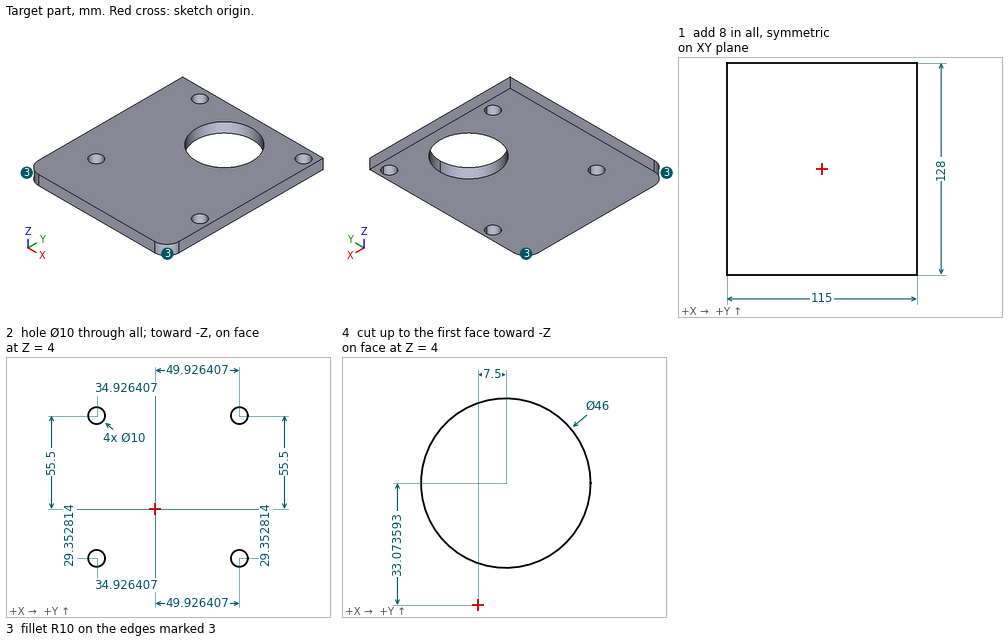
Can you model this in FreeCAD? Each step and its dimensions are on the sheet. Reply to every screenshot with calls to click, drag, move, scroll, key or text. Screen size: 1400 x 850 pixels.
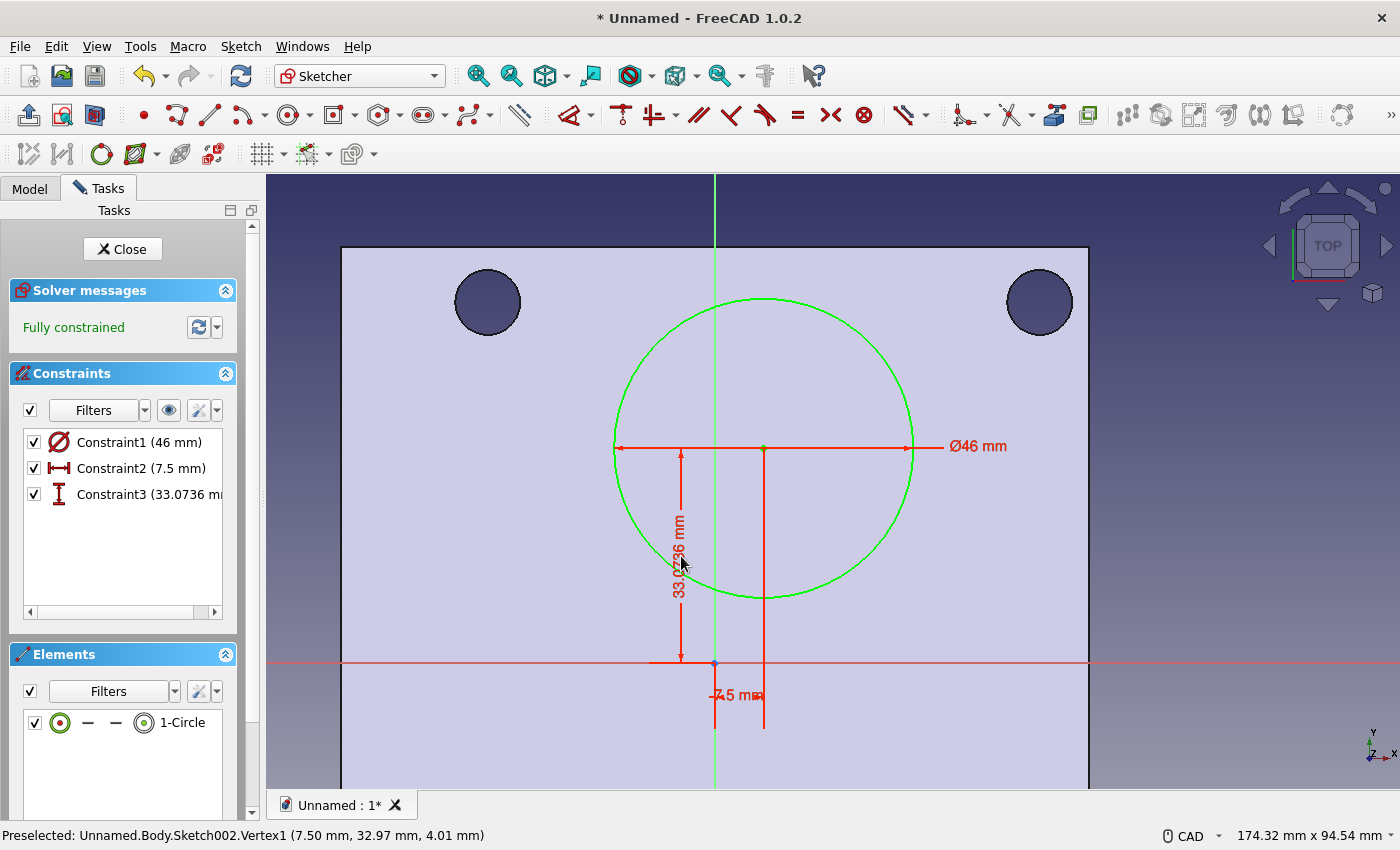
click(123, 249)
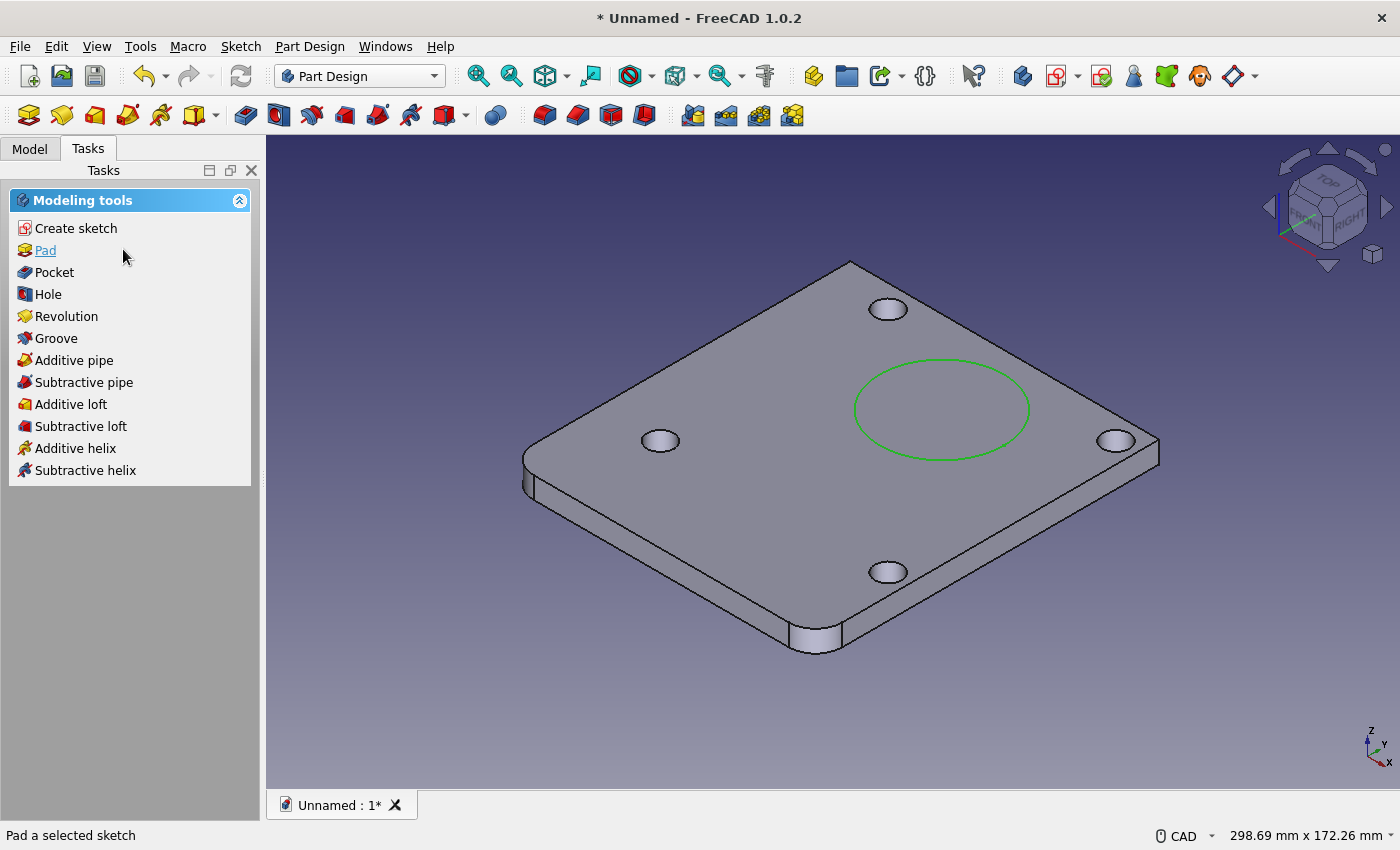
click(246, 116)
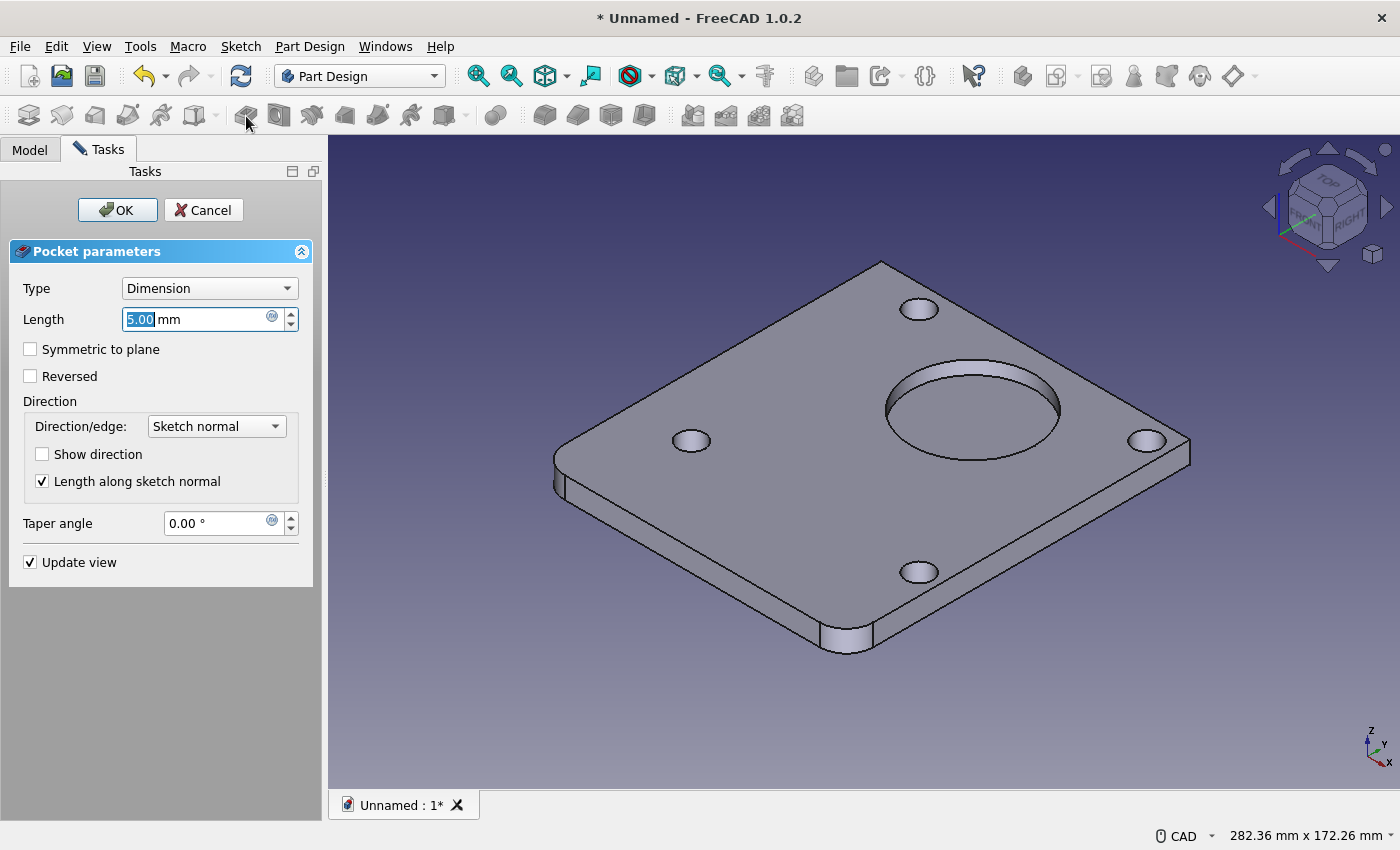
click(210, 288)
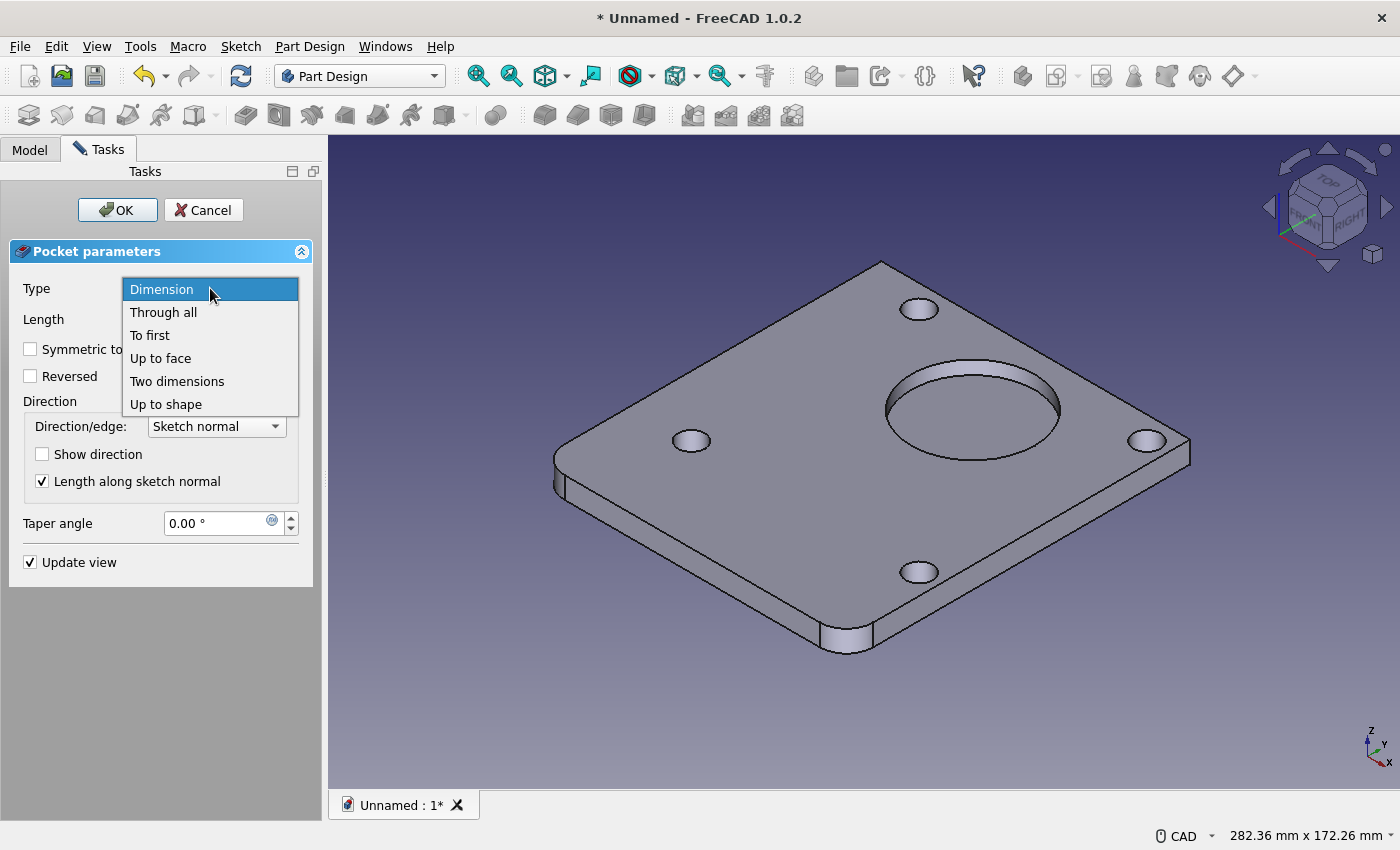
click(208, 336)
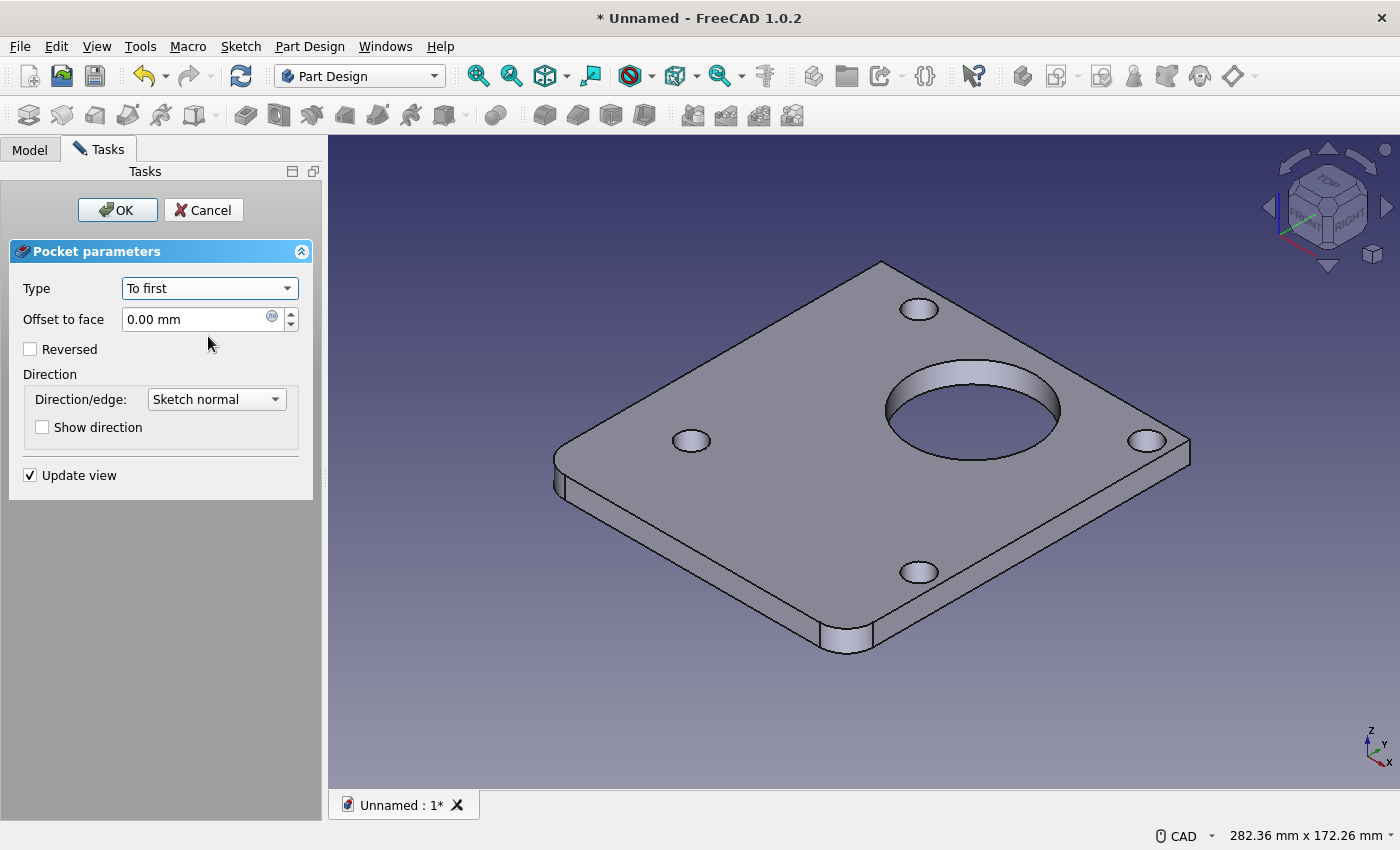
click(118, 210)